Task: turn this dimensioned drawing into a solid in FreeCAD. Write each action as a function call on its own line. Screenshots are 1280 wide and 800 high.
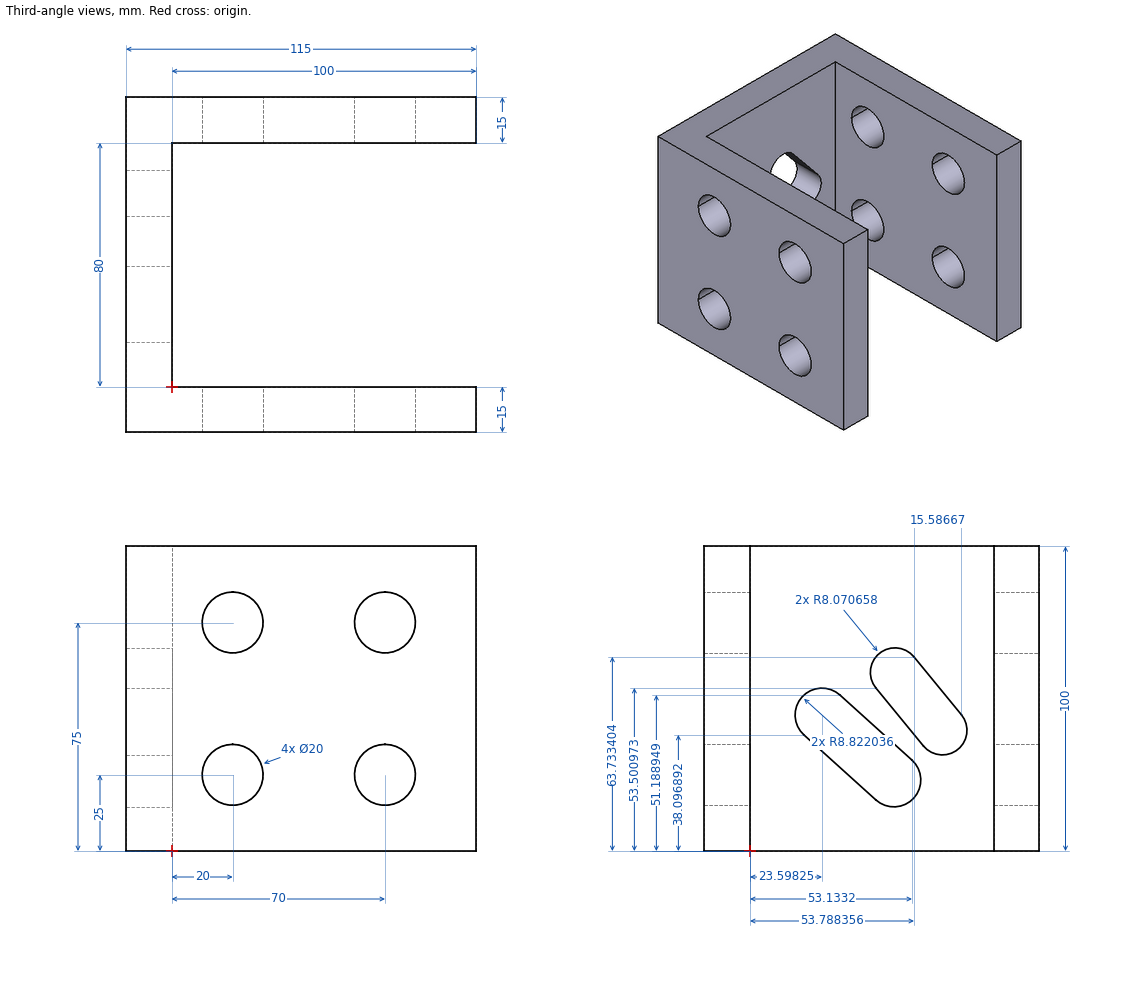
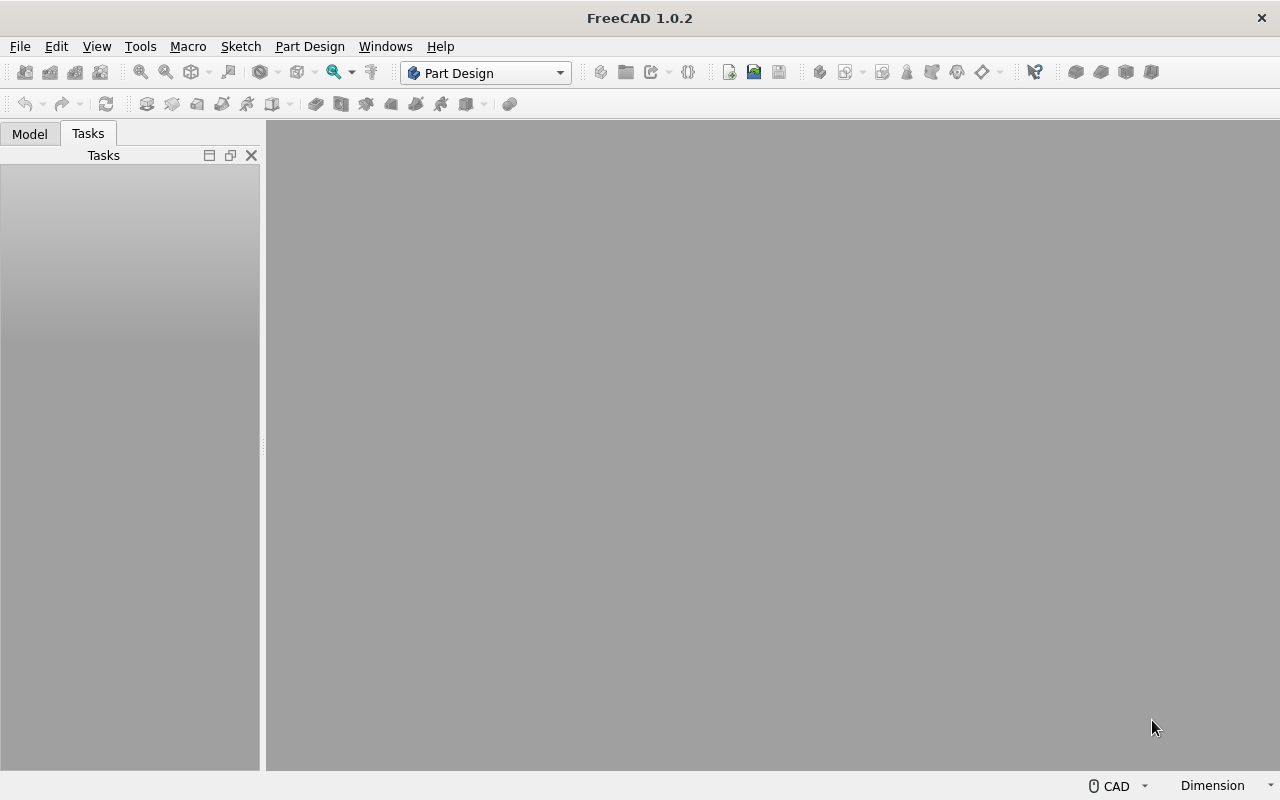
click(729, 72)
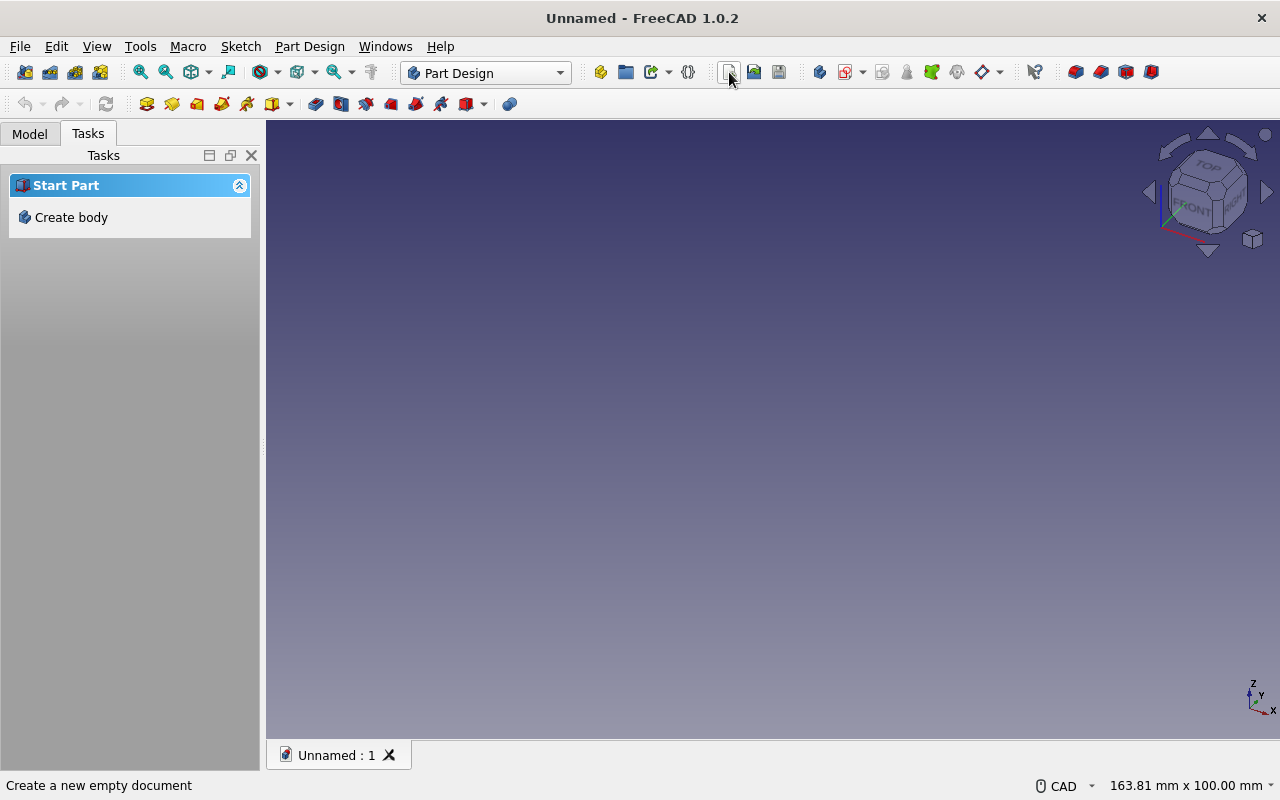
click(844, 72)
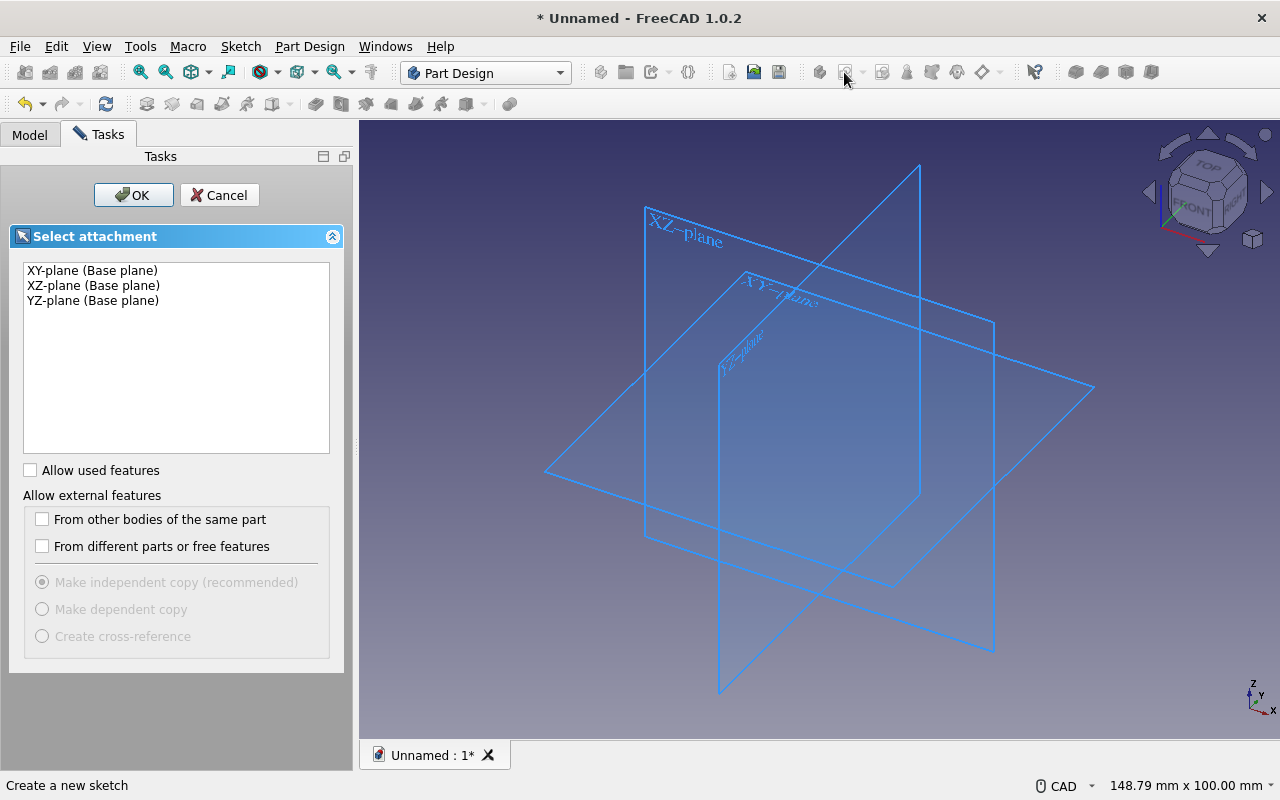
click(84, 270)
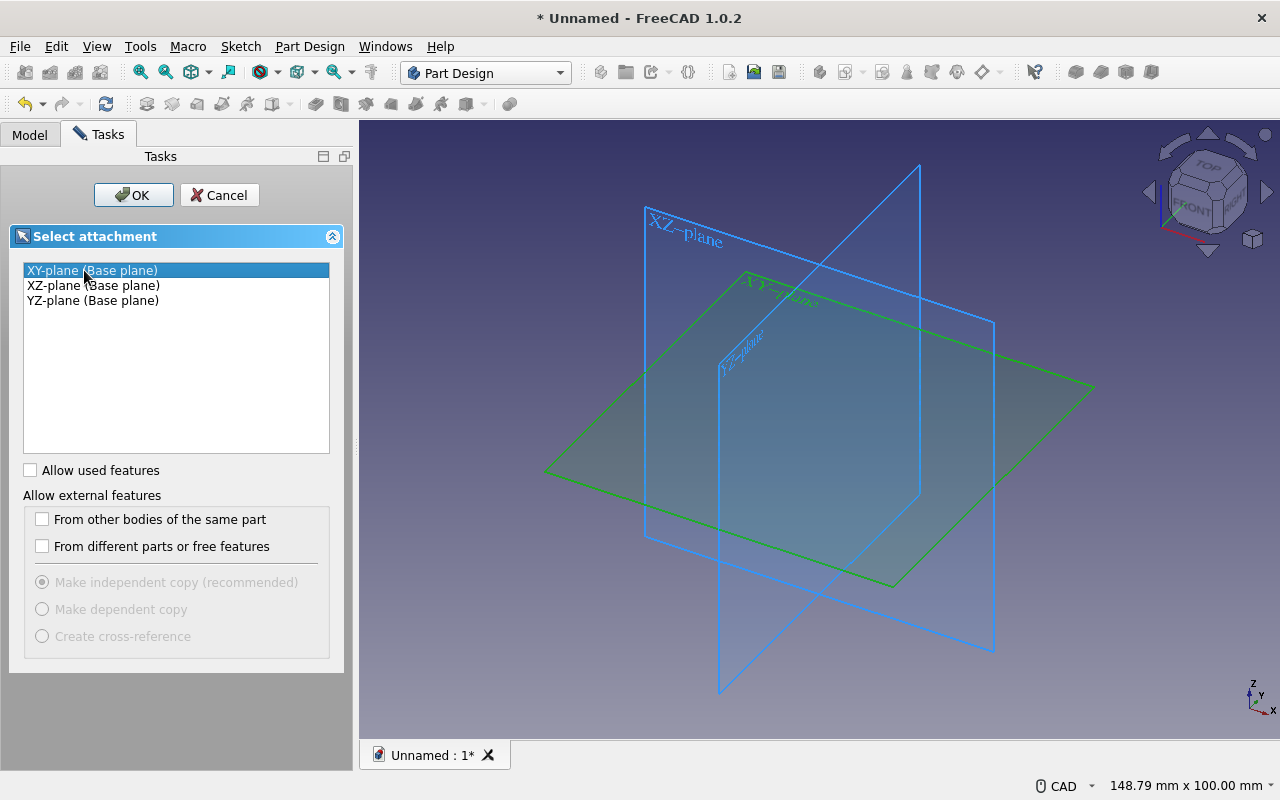
click(134, 195)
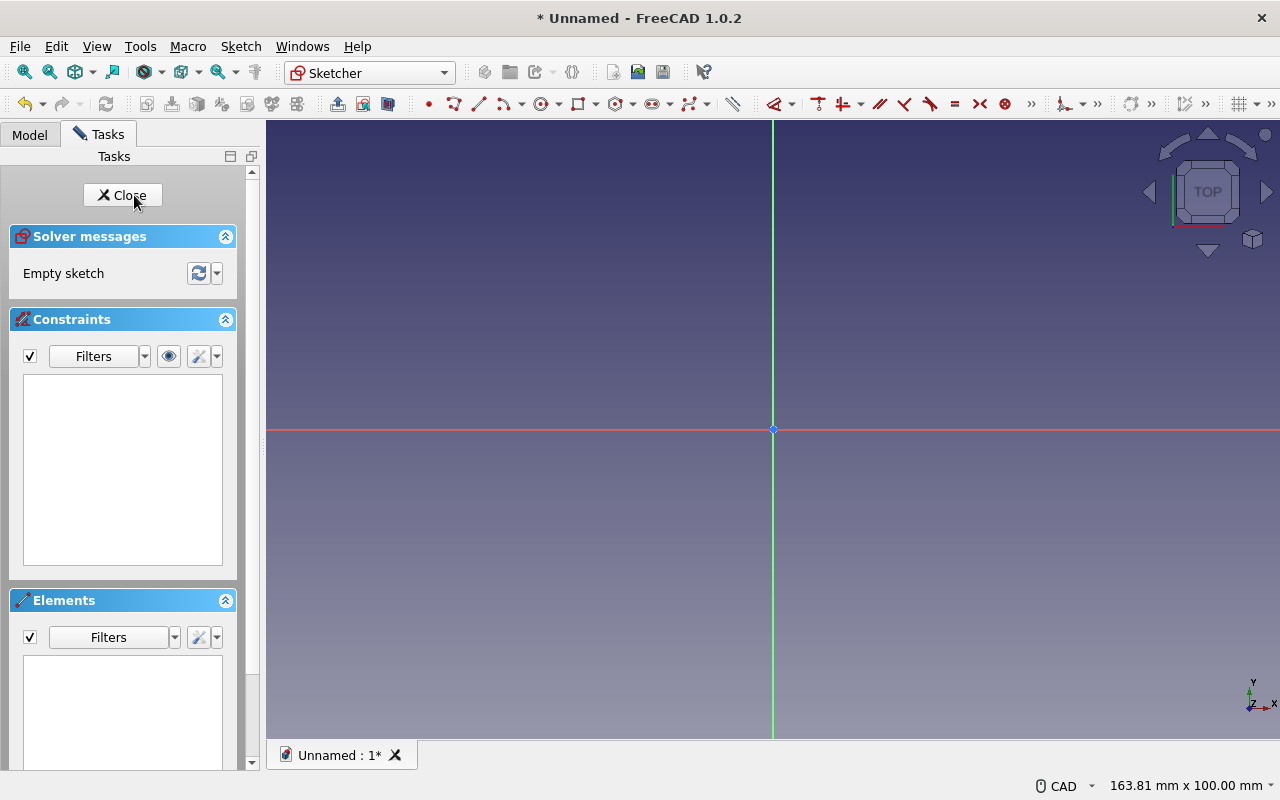
scroll(301, 711, down, 3)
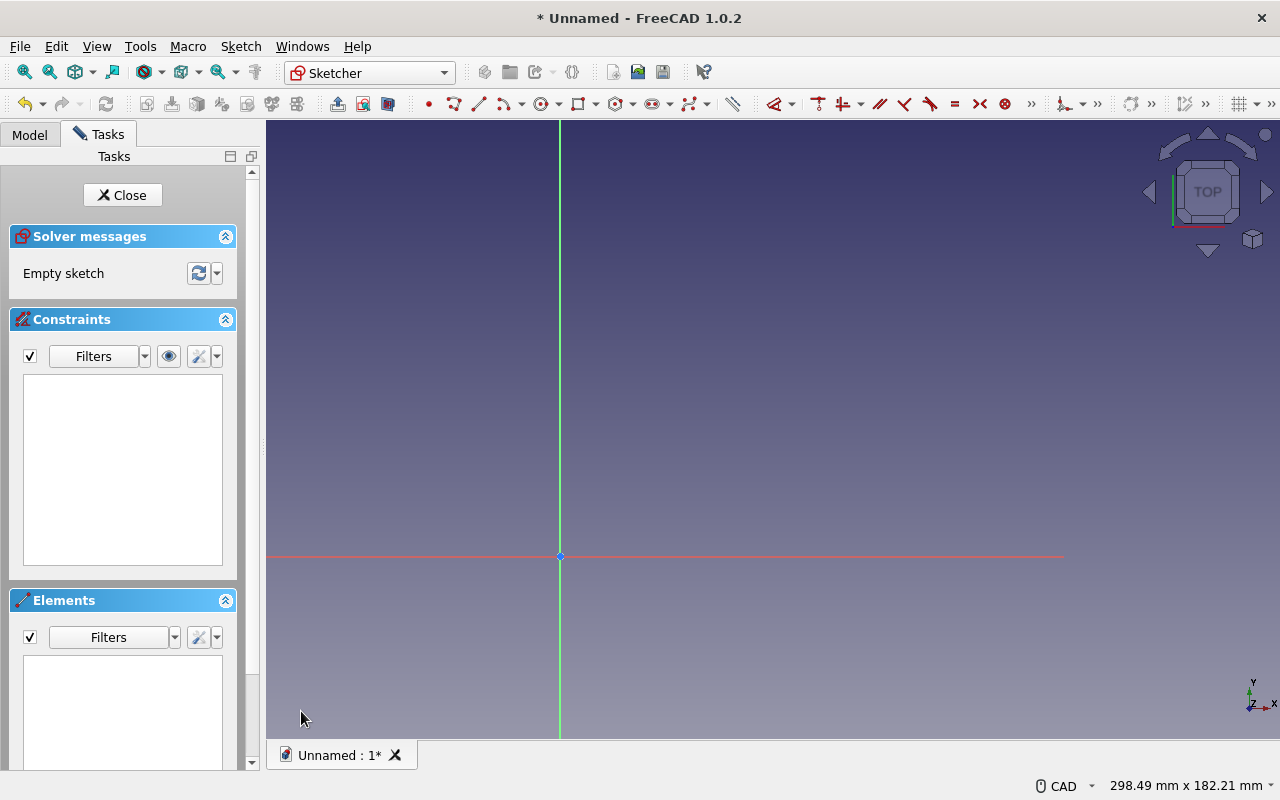
click(454, 104)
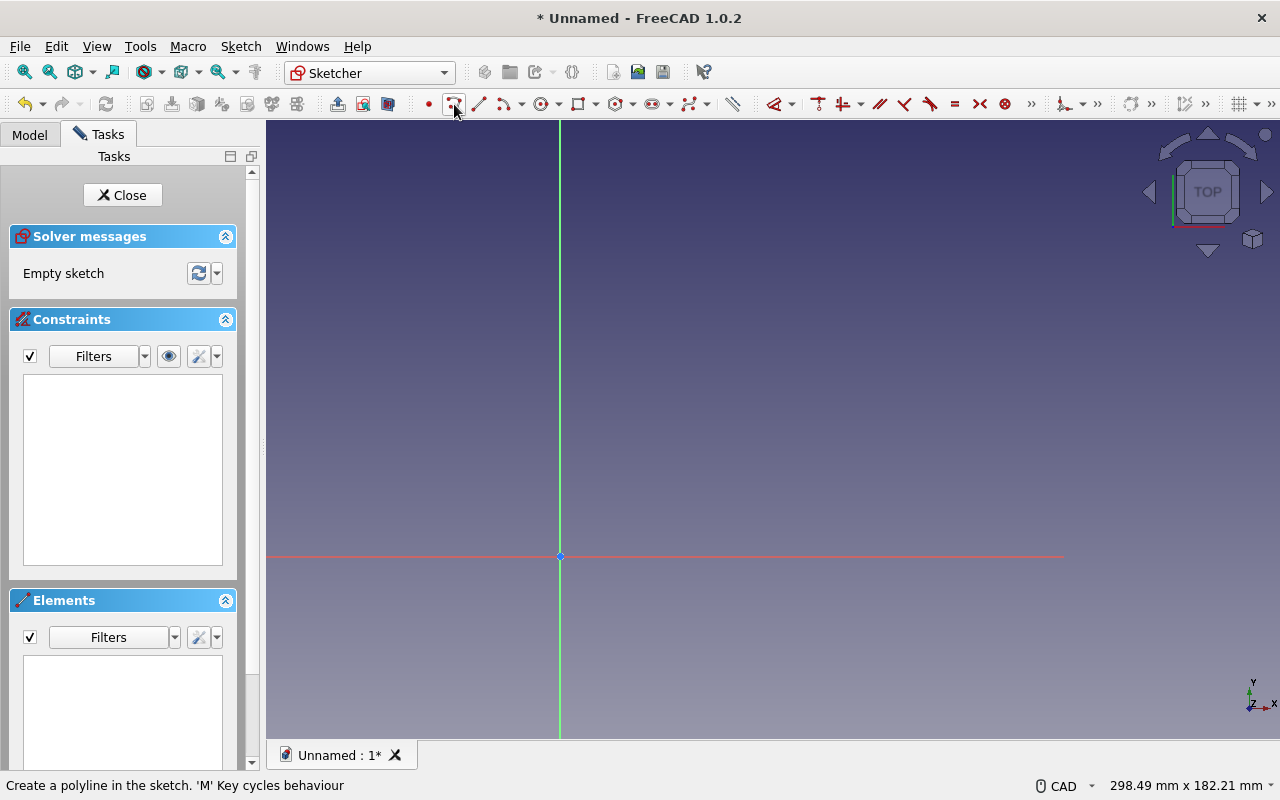
click(560, 557)
click(569, 285)
click(900, 285)
click(900, 234)
click(509, 234)
click(509, 608)
click(900, 608)
click(900, 548)
click(560, 557)
key(Escape)
key(Escape)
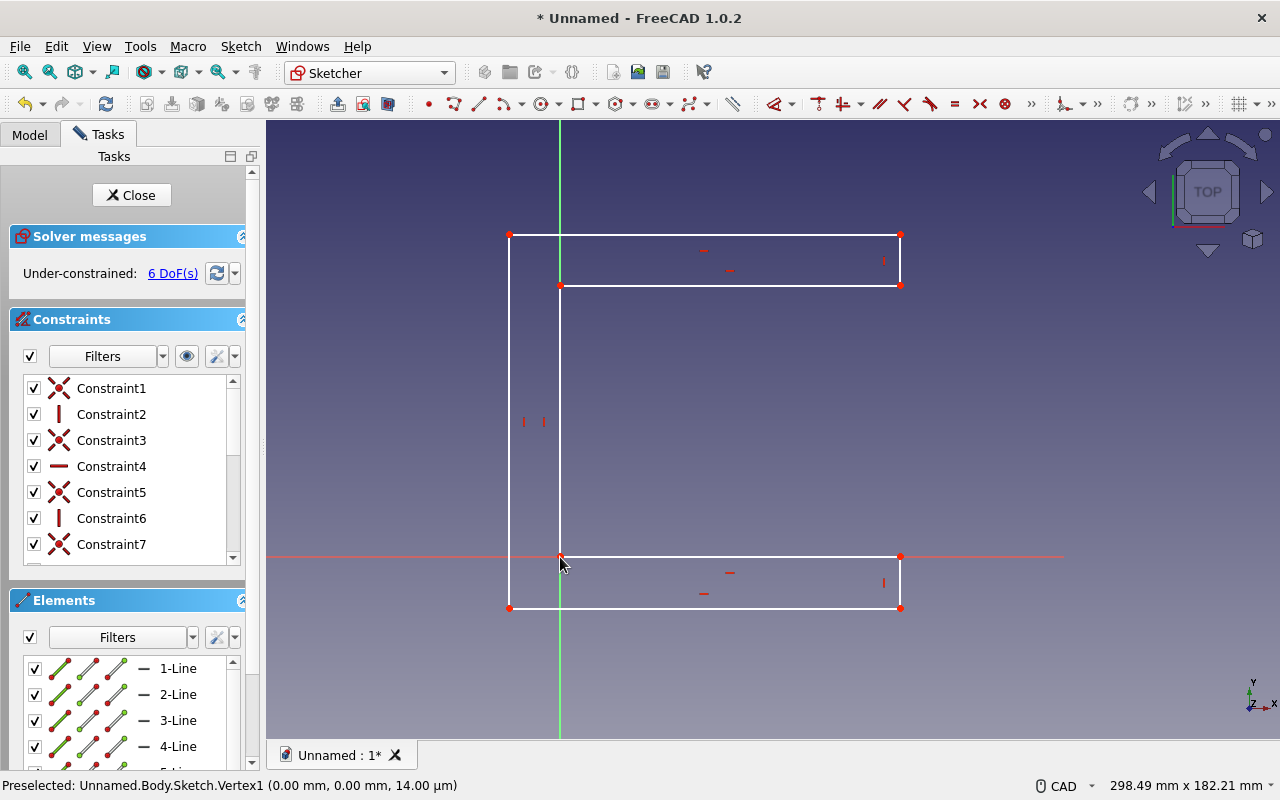
click(774, 104)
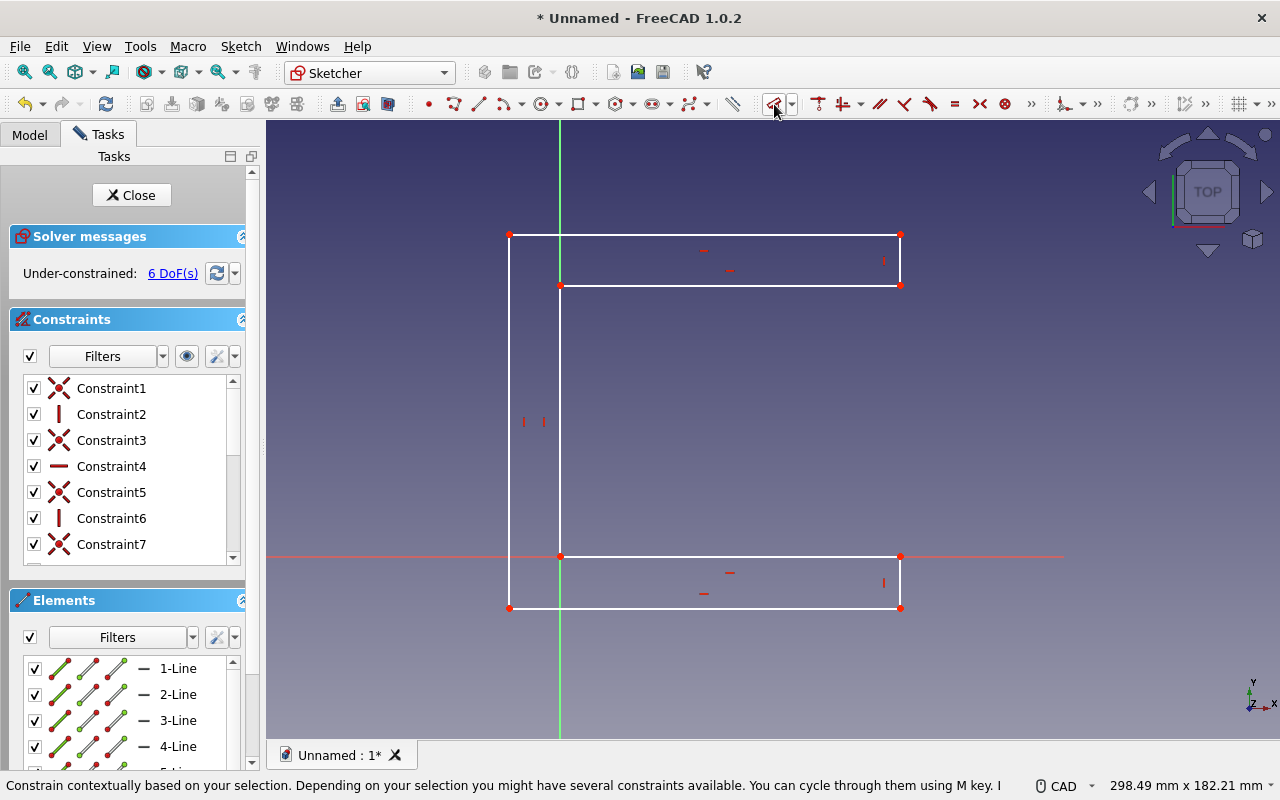
click(560, 476)
click(526, 421)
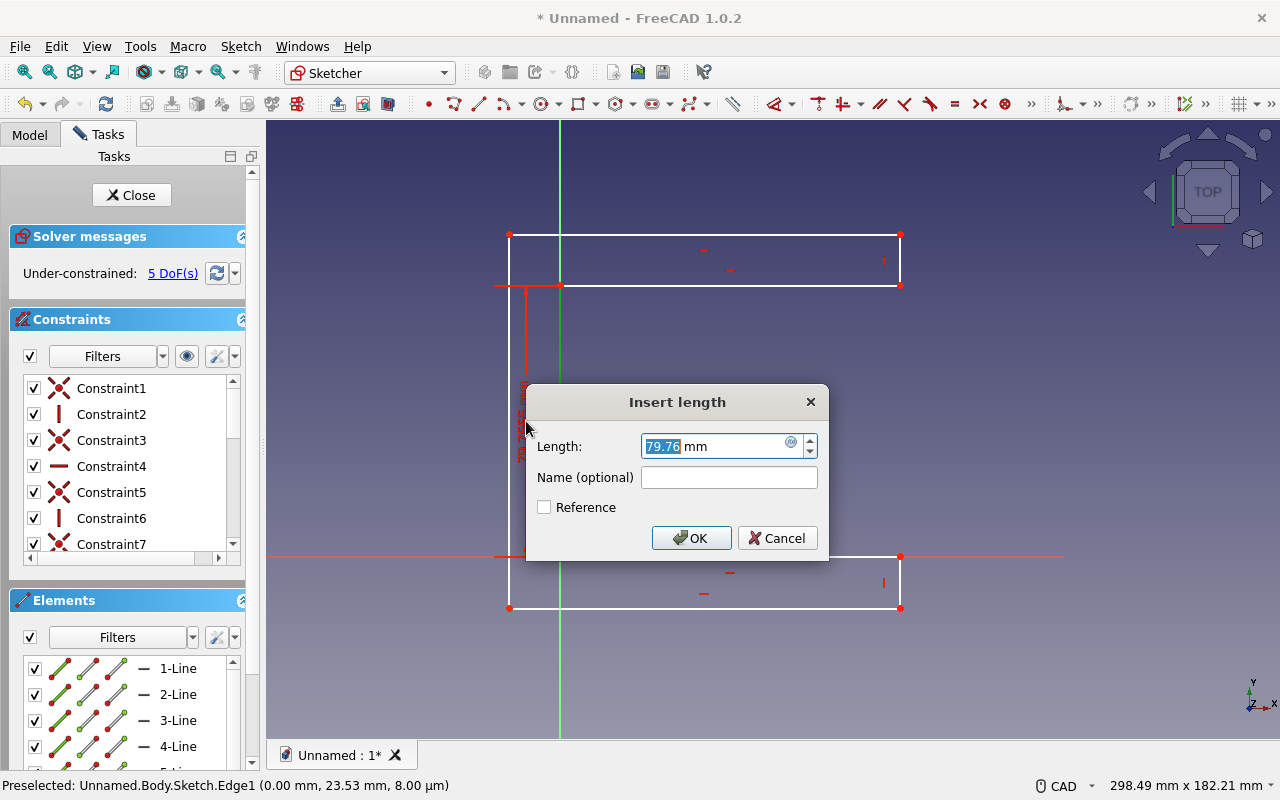
text(80)
key(Return)